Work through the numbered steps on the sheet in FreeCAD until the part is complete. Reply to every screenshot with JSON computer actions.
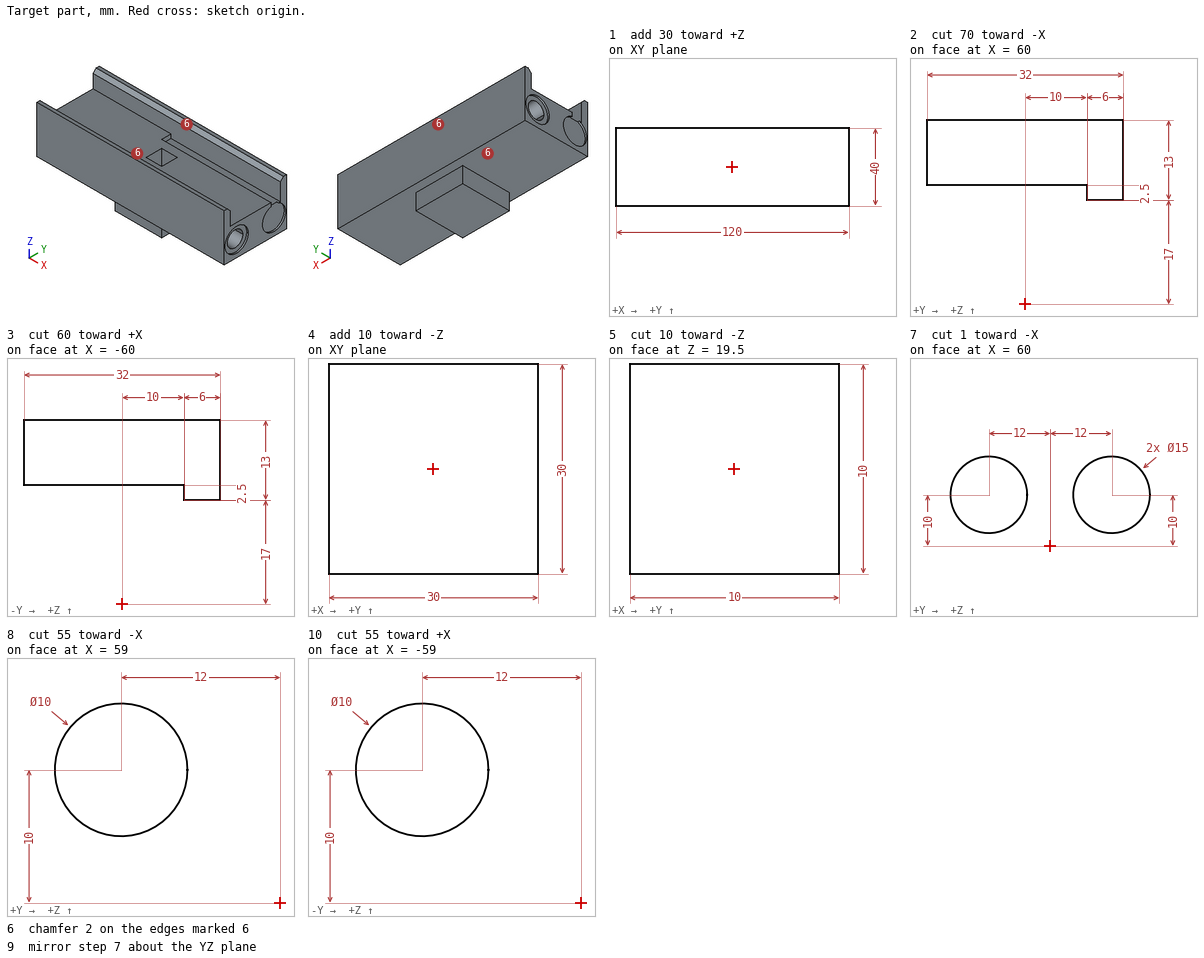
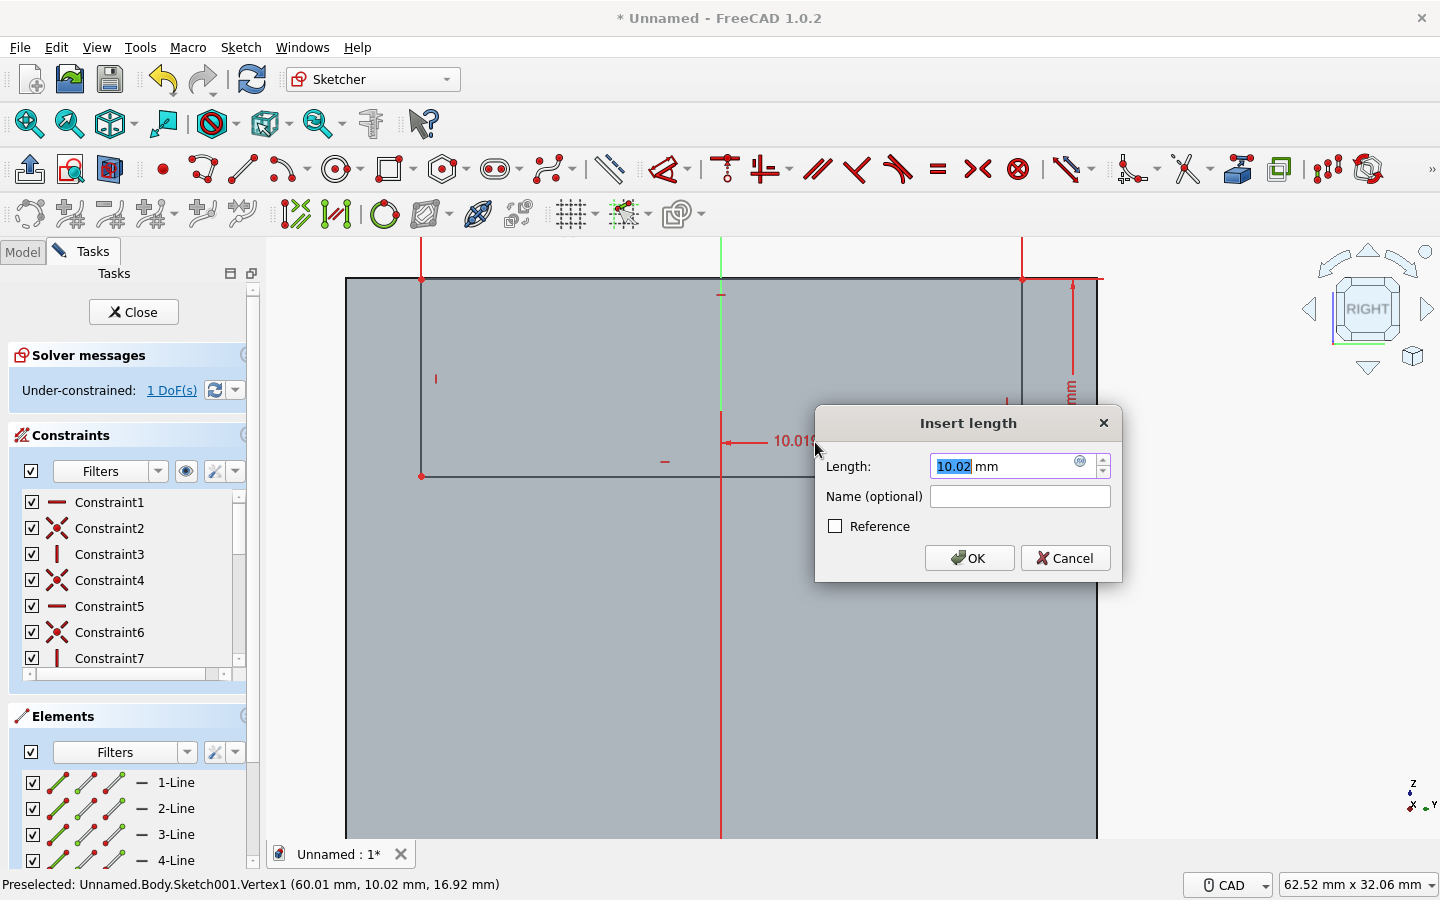
{"action": "type", "text": "10"}
{"action": "key", "text": "Return"}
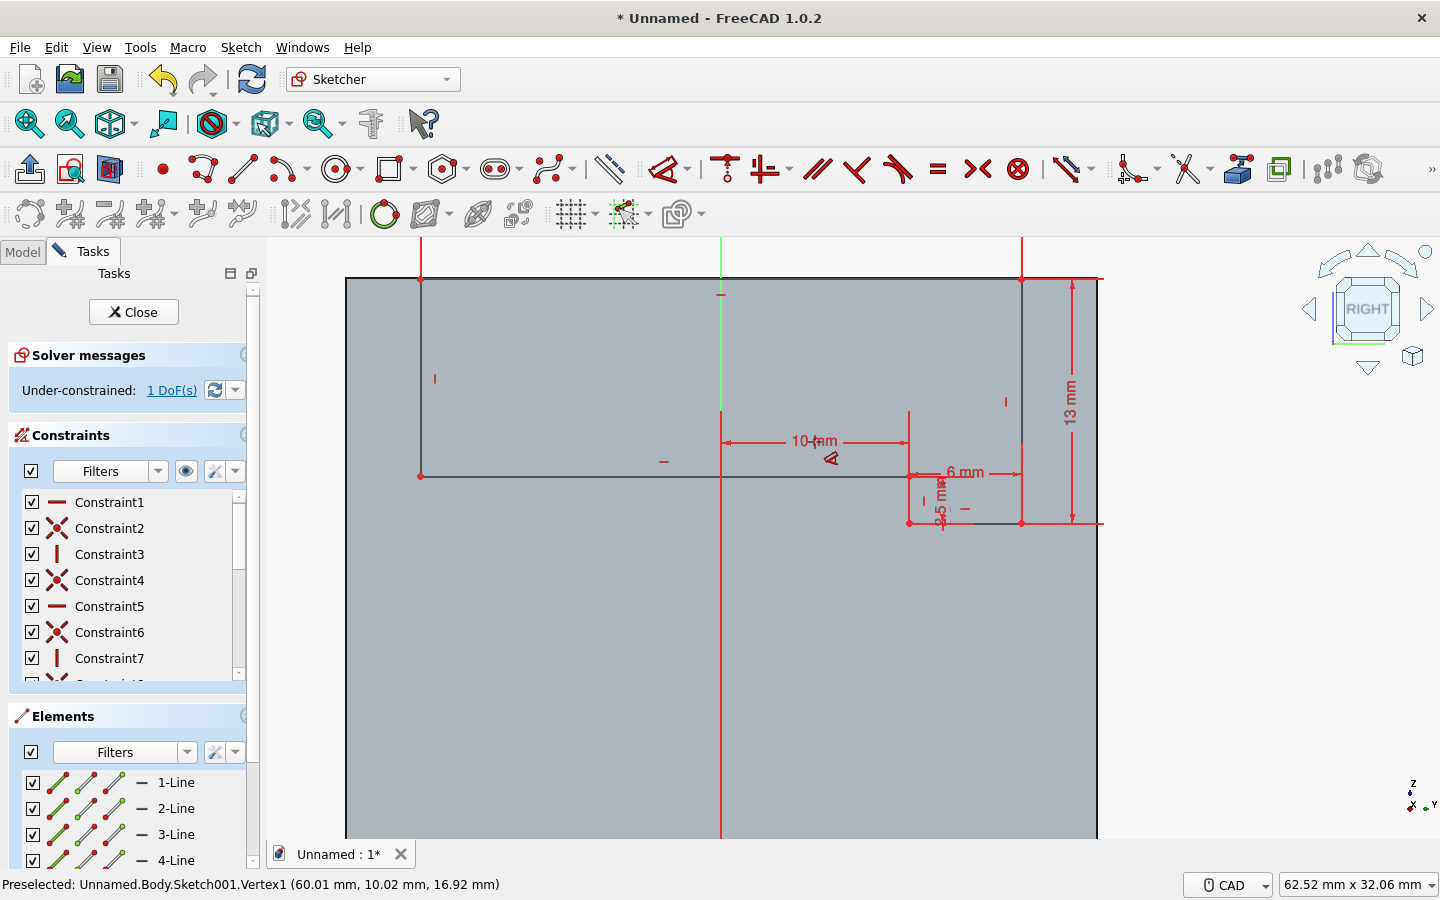
{"action": "left_click", "coordinate": [909, 524]}
{"action": "left_click", "coordinate": [943, 667]}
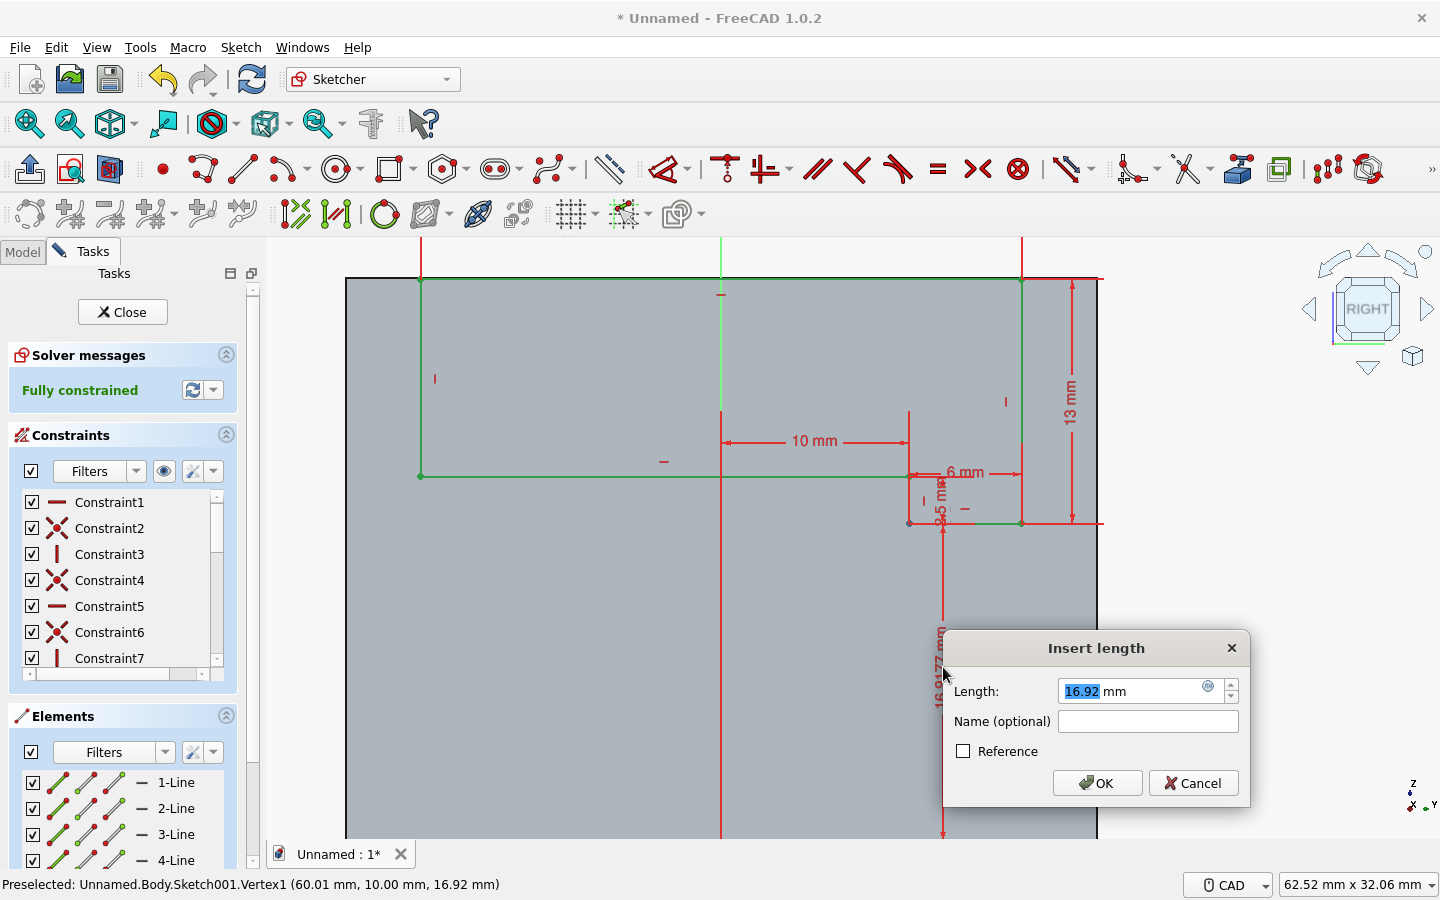
{"action": "type", "text": "17"}
{"action": "key", "text": "Return"}
{"action": "key", "text": "Escape"}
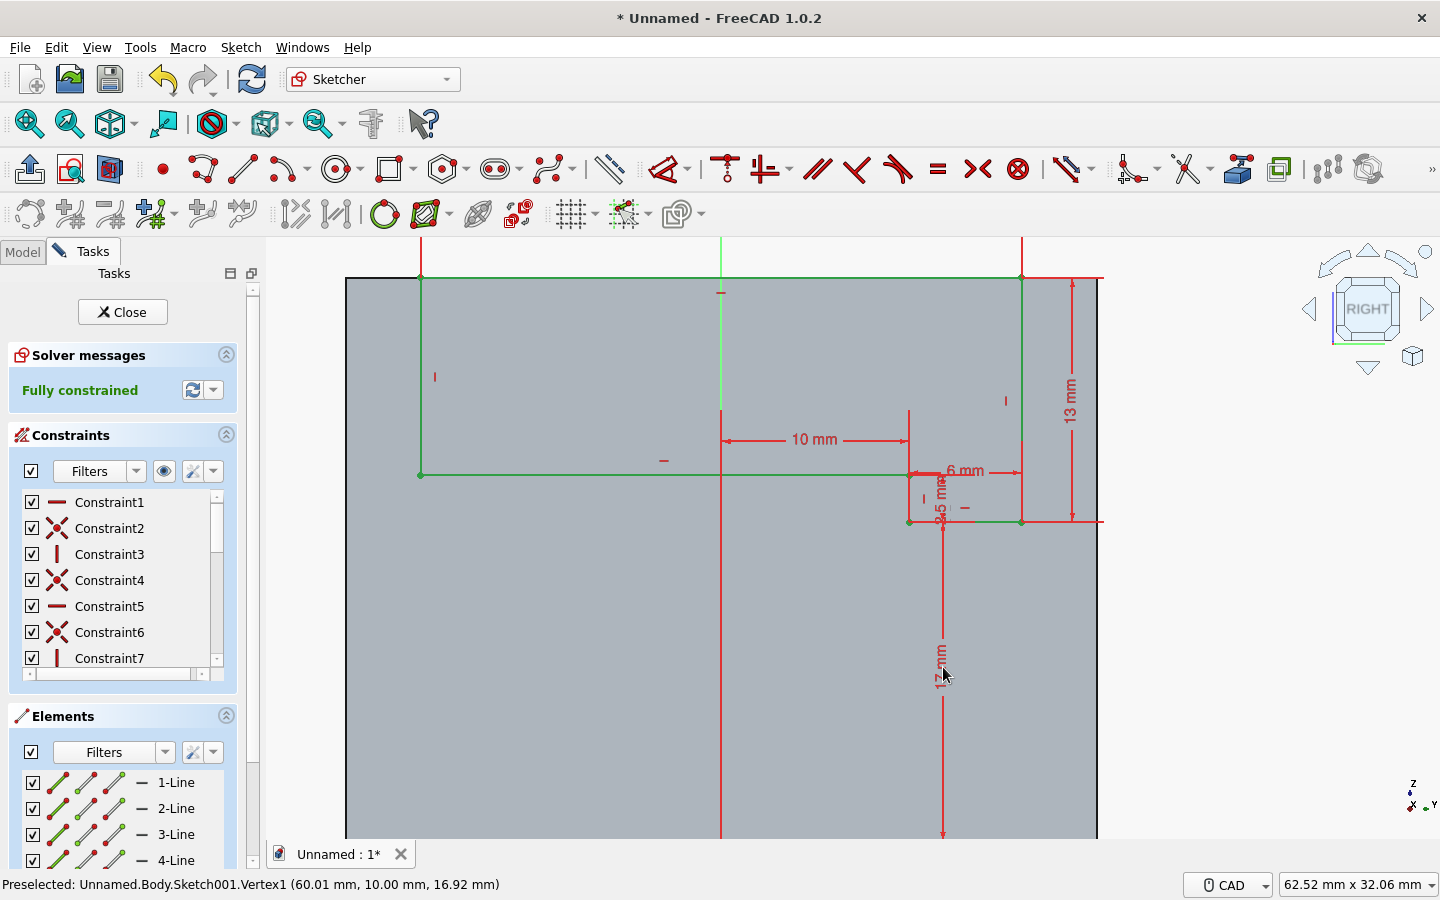
{"action": "left_click", "coordinate": [123, 312]}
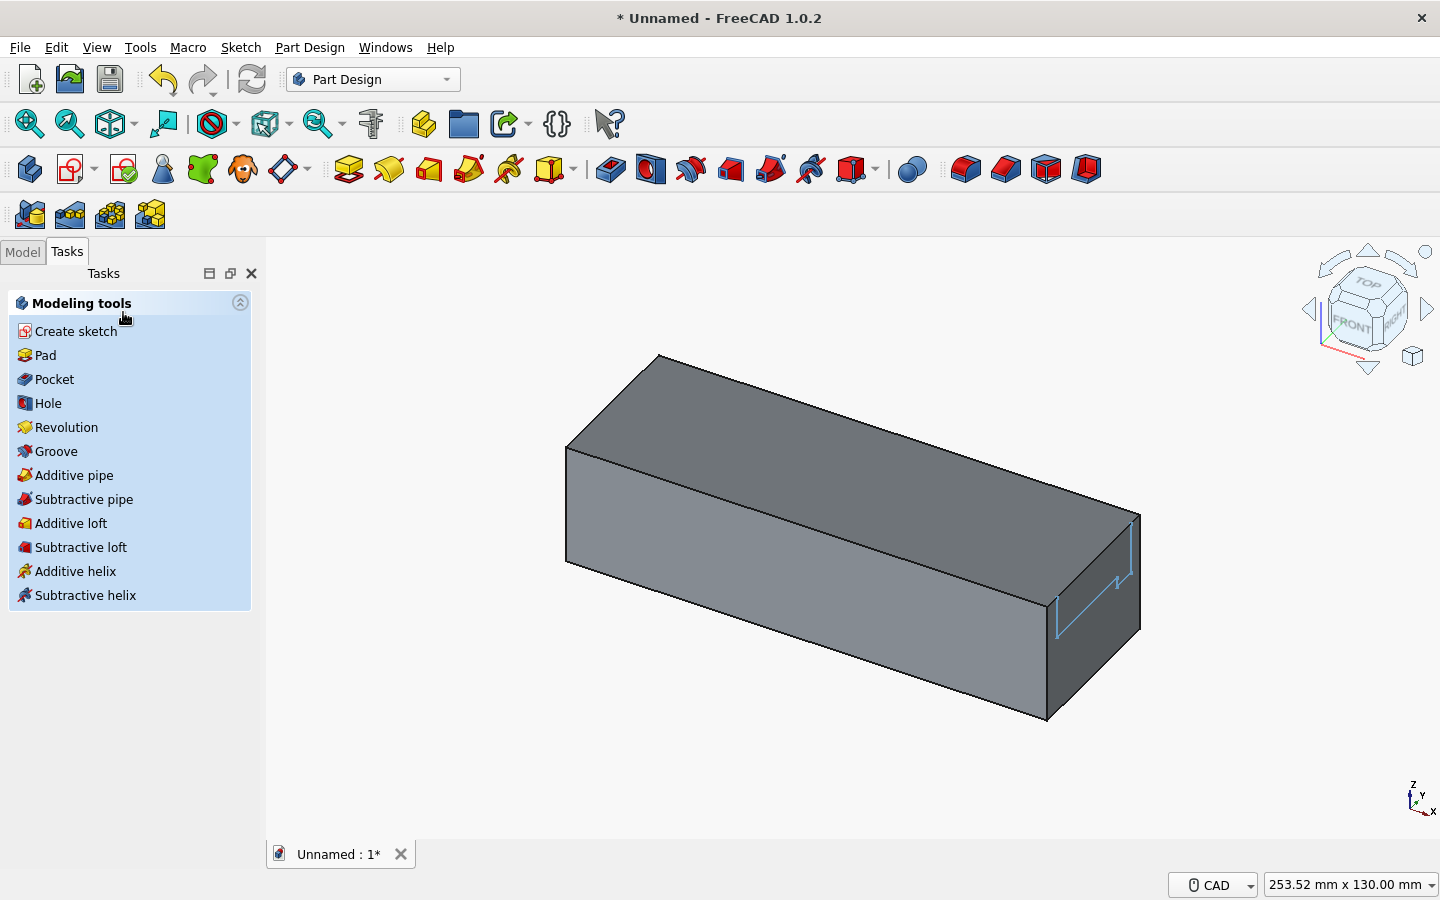
{"action": "left_click", "coordinate": [612, 170]}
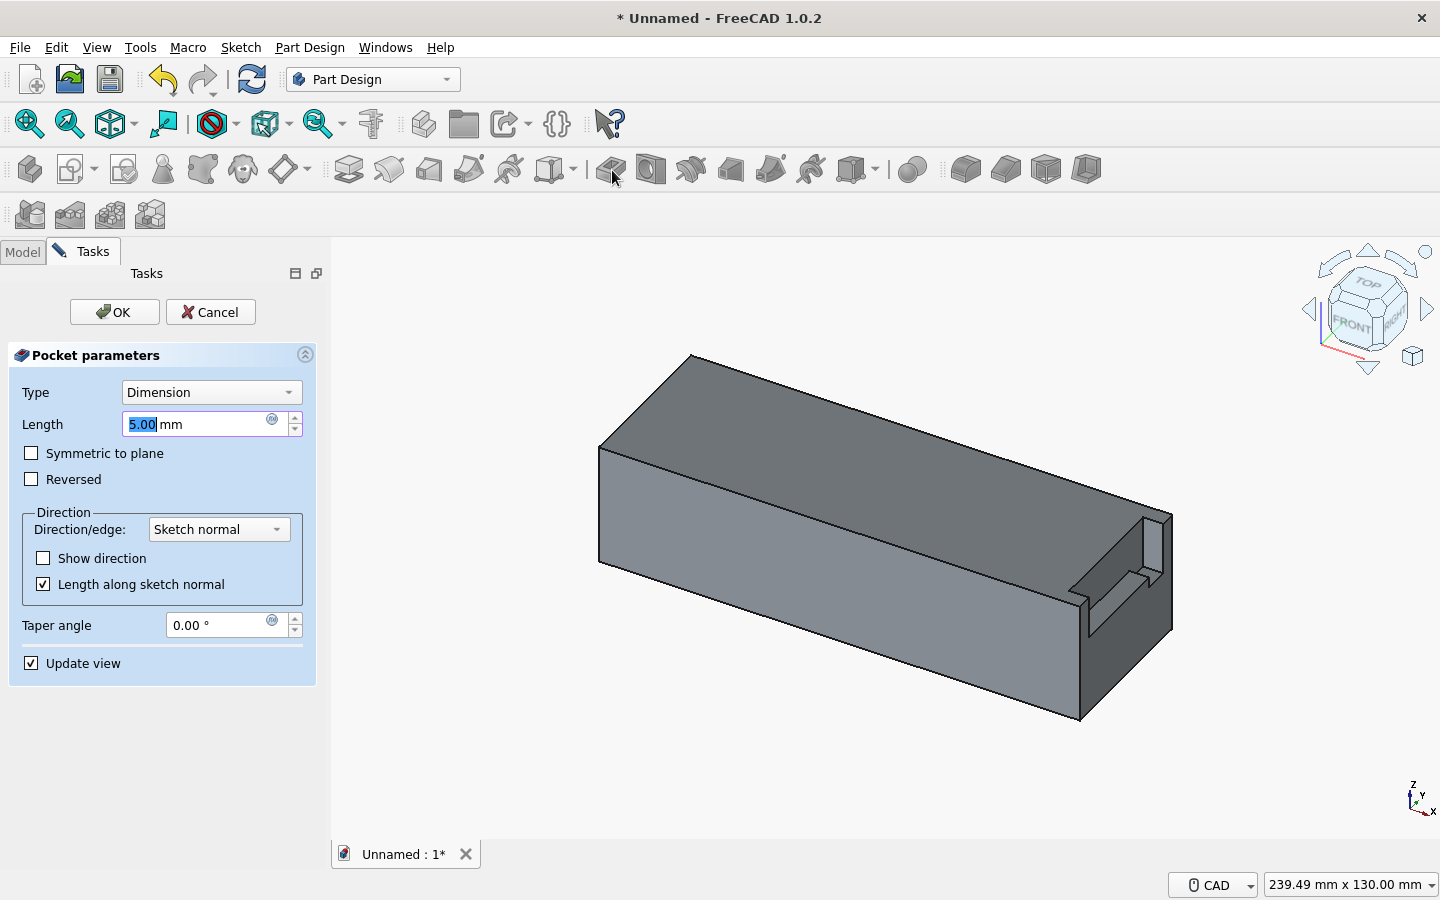
{"action": "type", "text": "70"}
{"action": "key", "text": "Tab"}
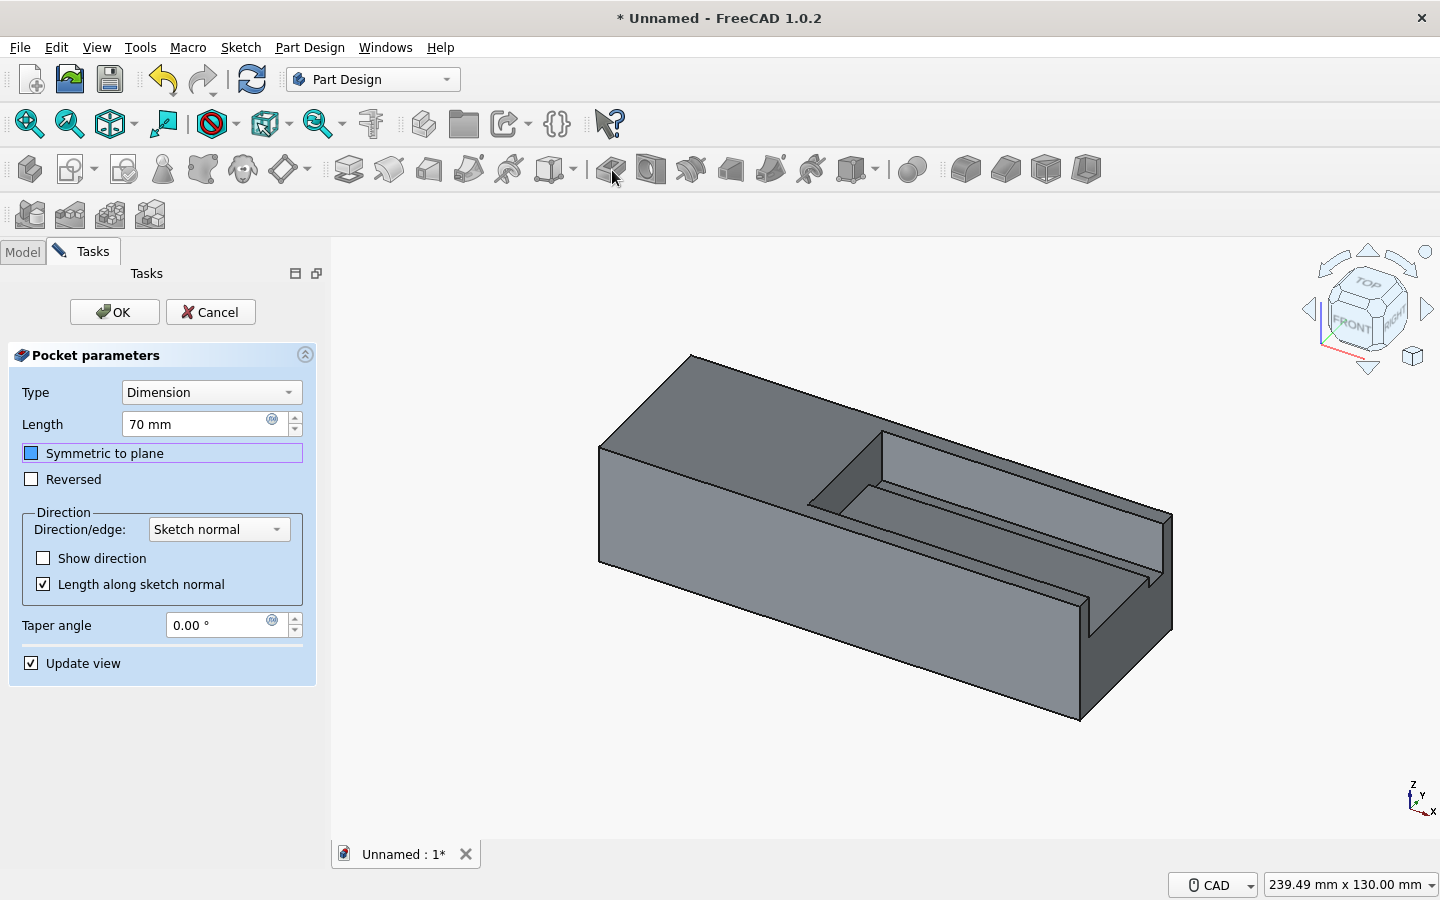
{"action": "left_click", "coordinate": [115, 312]}